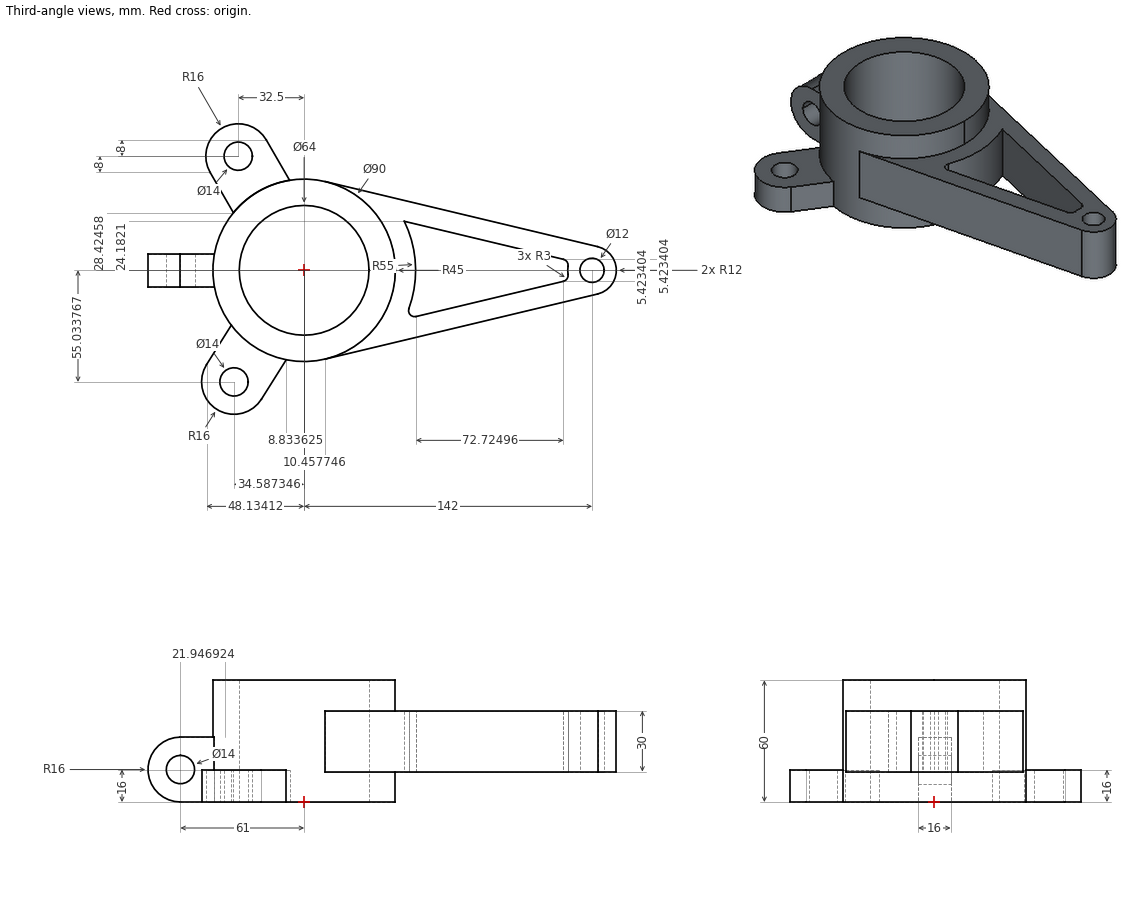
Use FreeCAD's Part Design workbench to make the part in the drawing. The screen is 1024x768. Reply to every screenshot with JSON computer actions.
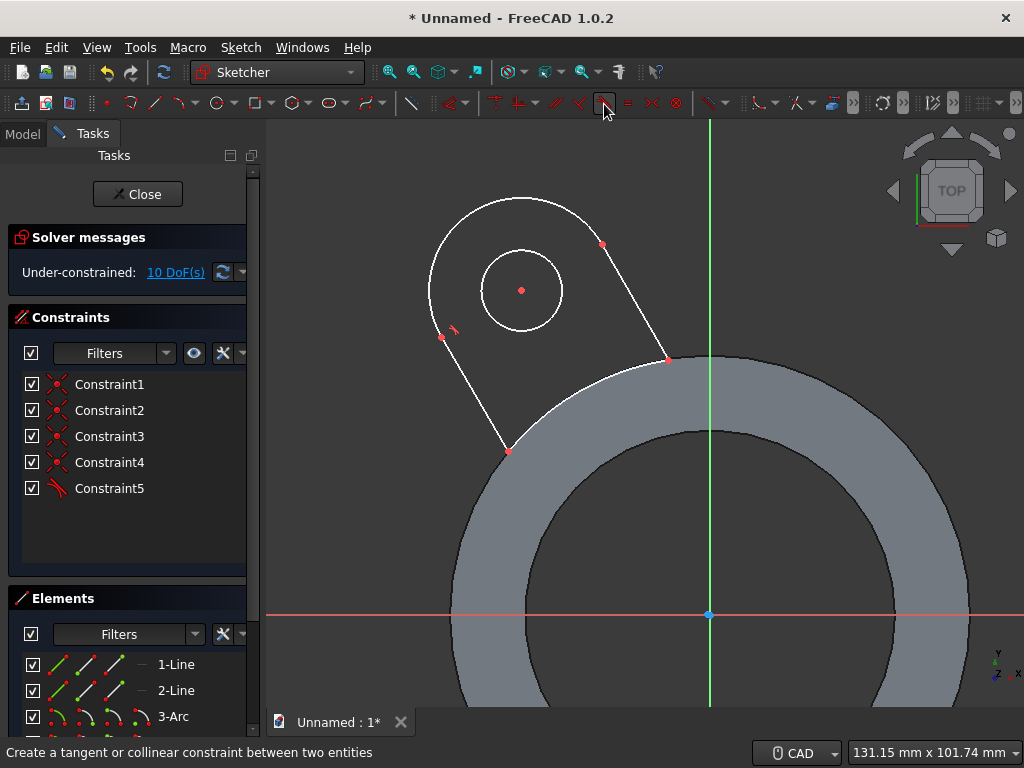
{"action": "left_click", "coordinate": [649, 325]}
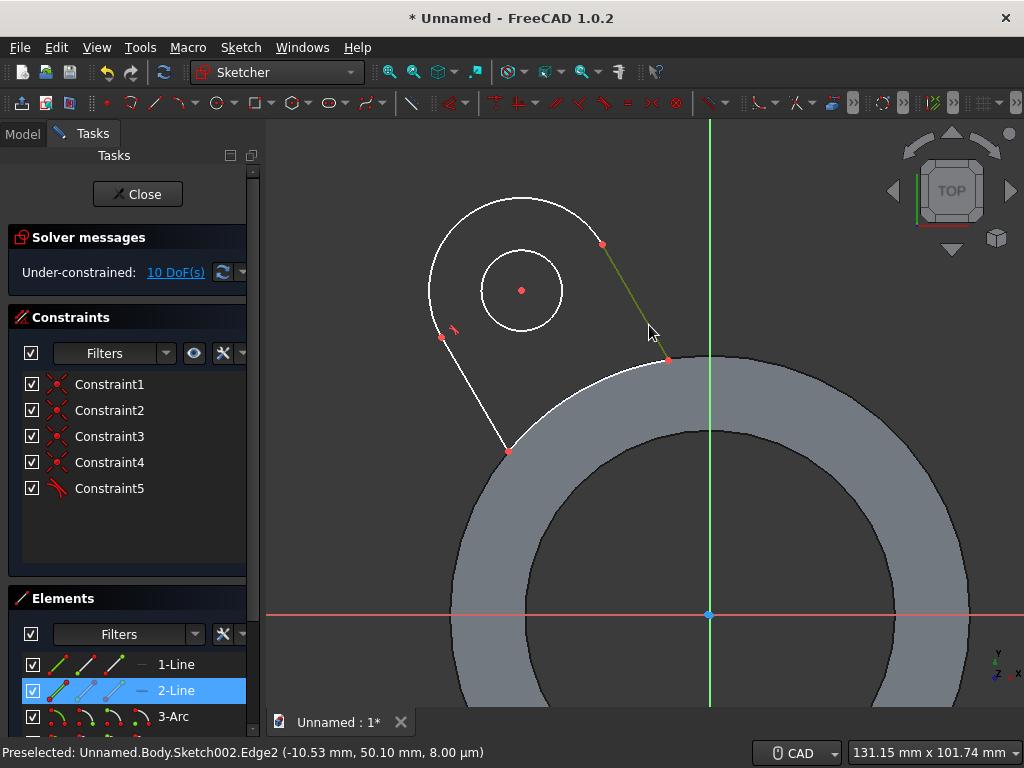
{"action": "left_click", "coordinate": [532, 198]}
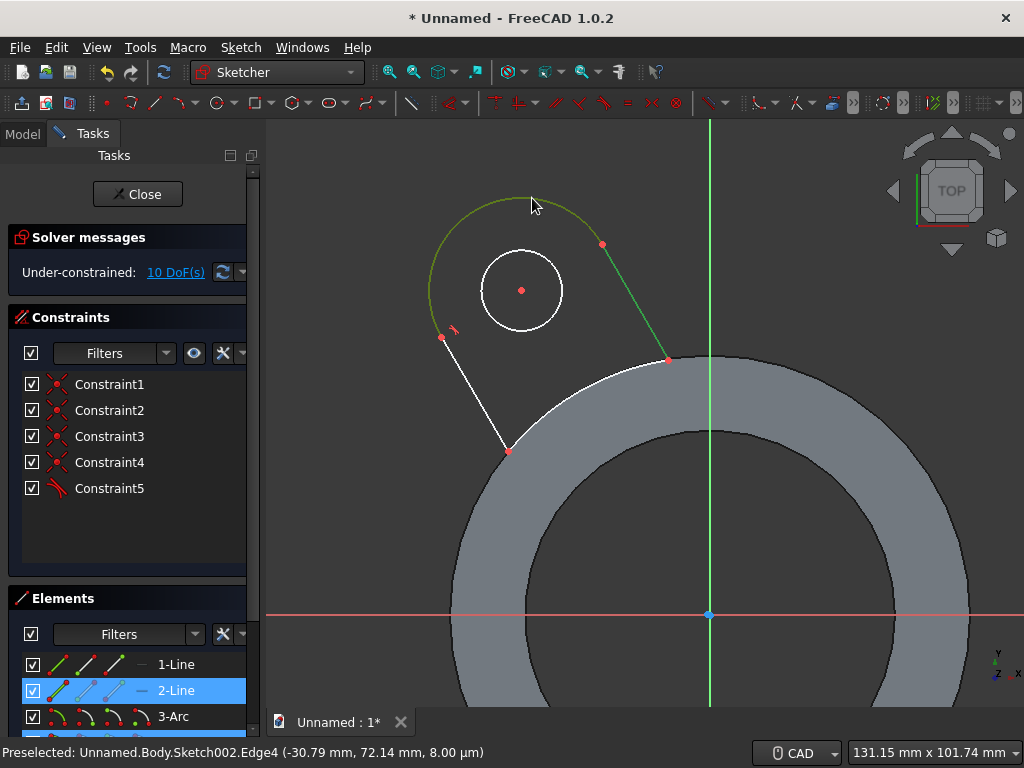
{"action": "key", "text": "t"}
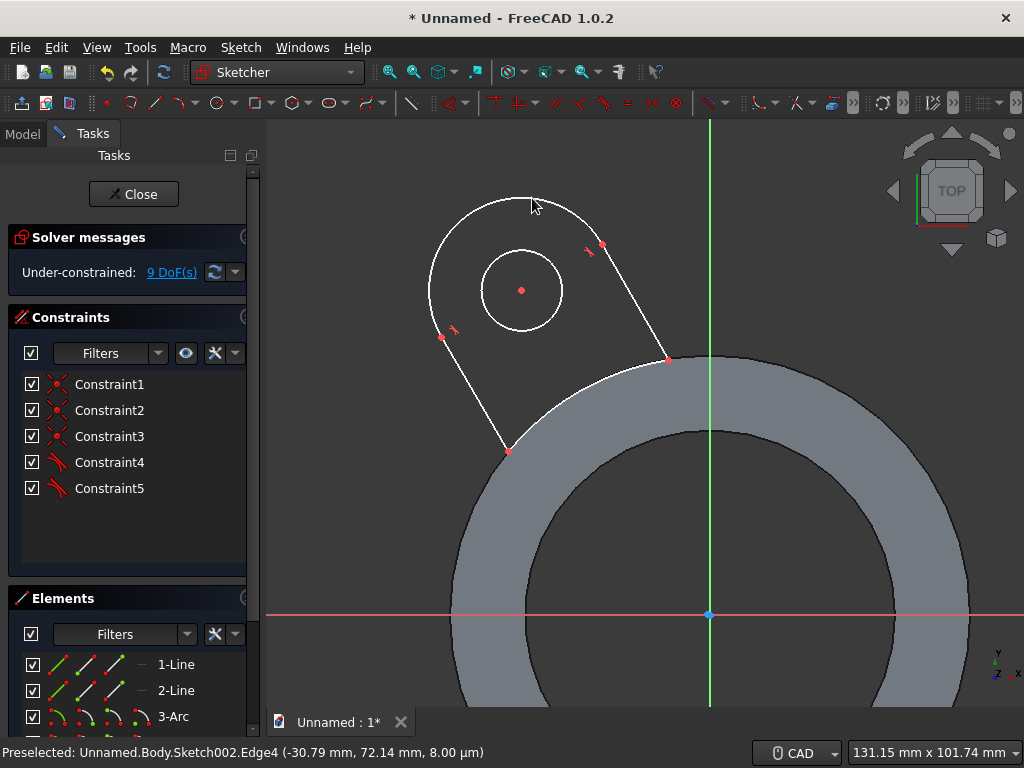
{"action": "left_click_drag", "start_coordinate": [698, 604], "coordinate": [720, 625]}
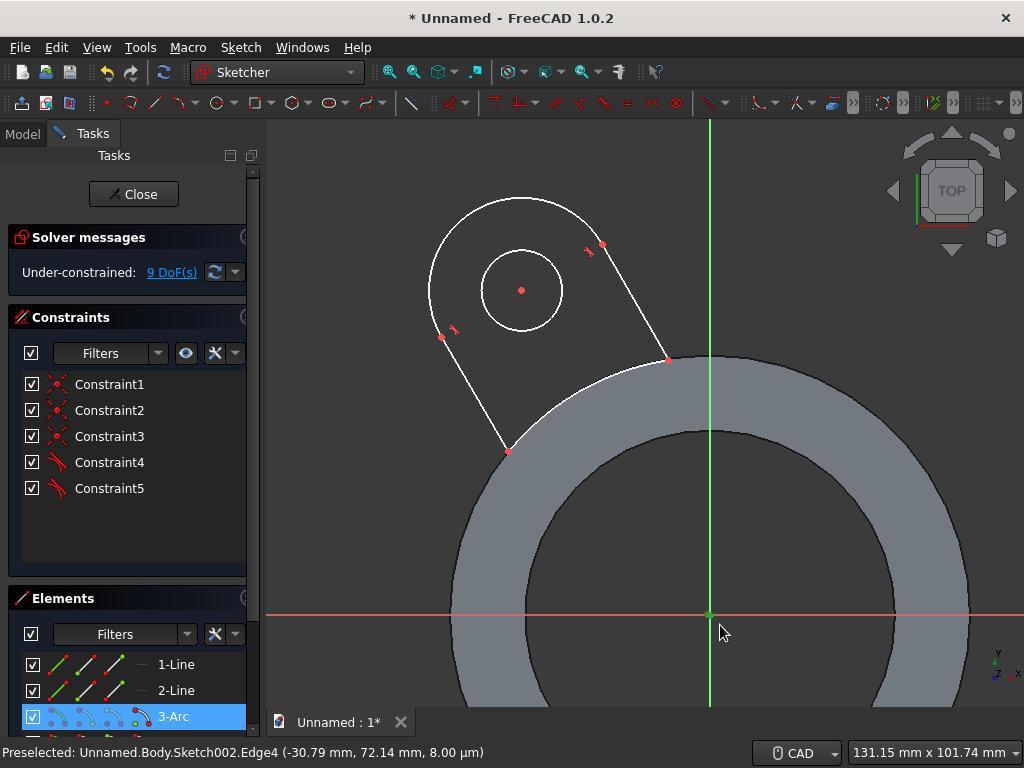
{"action": "left_click", "coordinate": [496, 104]}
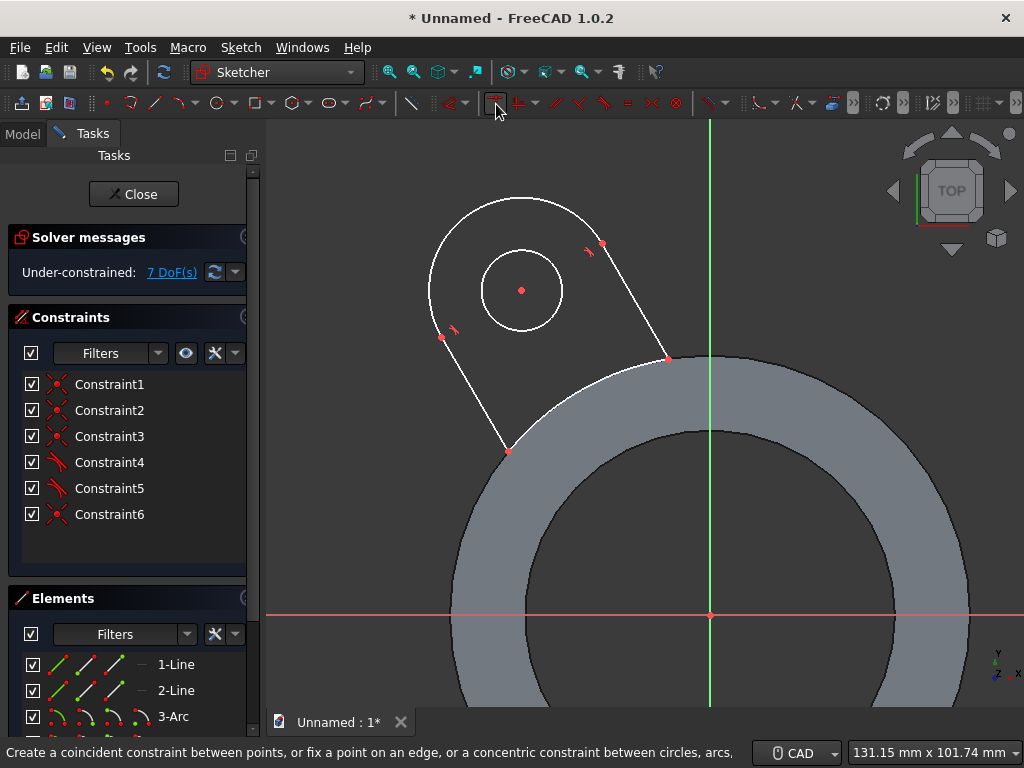
{"action": "left_click", "coordinate": [450, 104]}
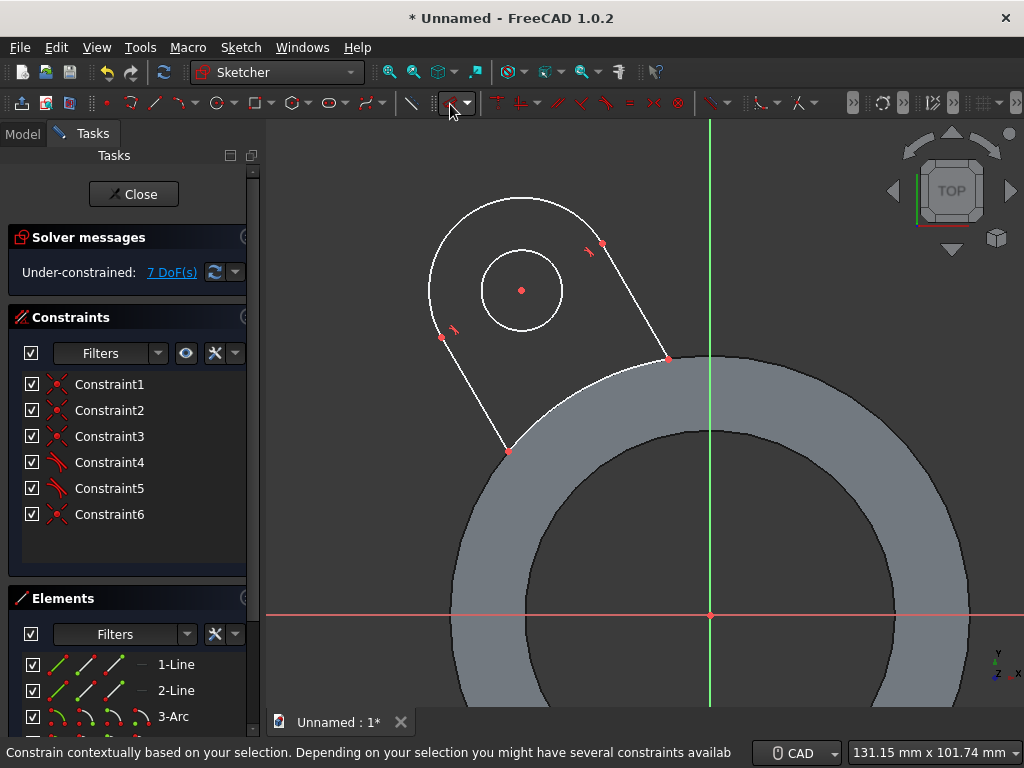
{"action": "left_click", "coordinate": [614, 374]}
{"action": "left_click", "coordinate": [602, 344]}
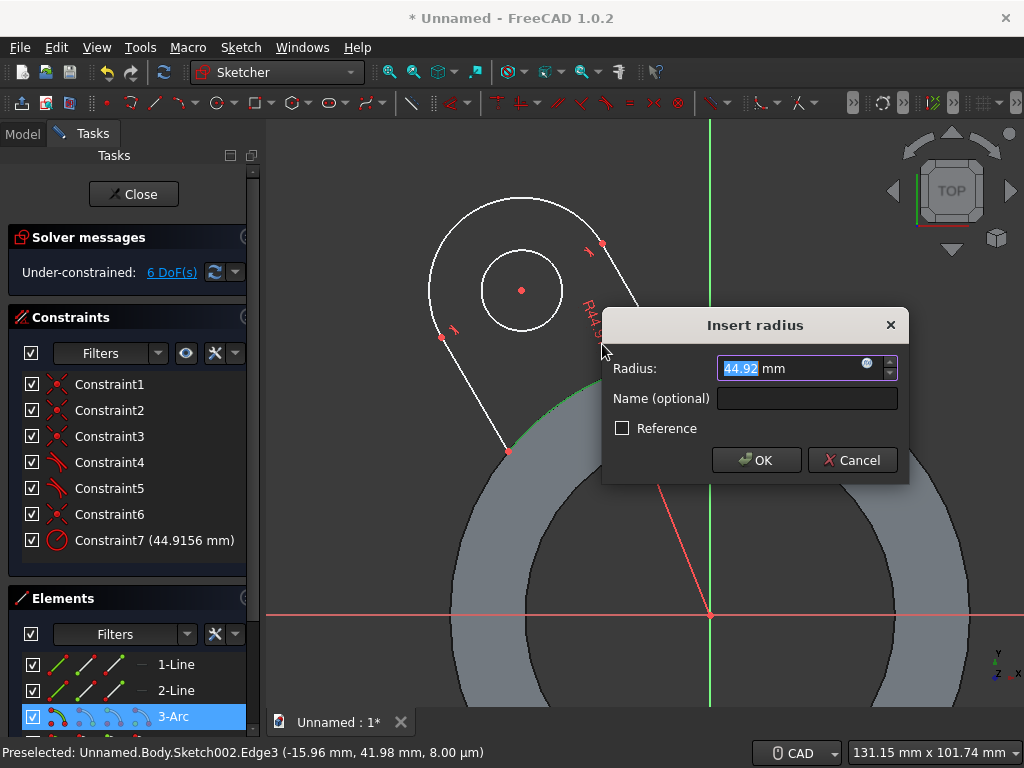
{"action": "type", "text": "45"}
{"action": "key", "text": "Return"}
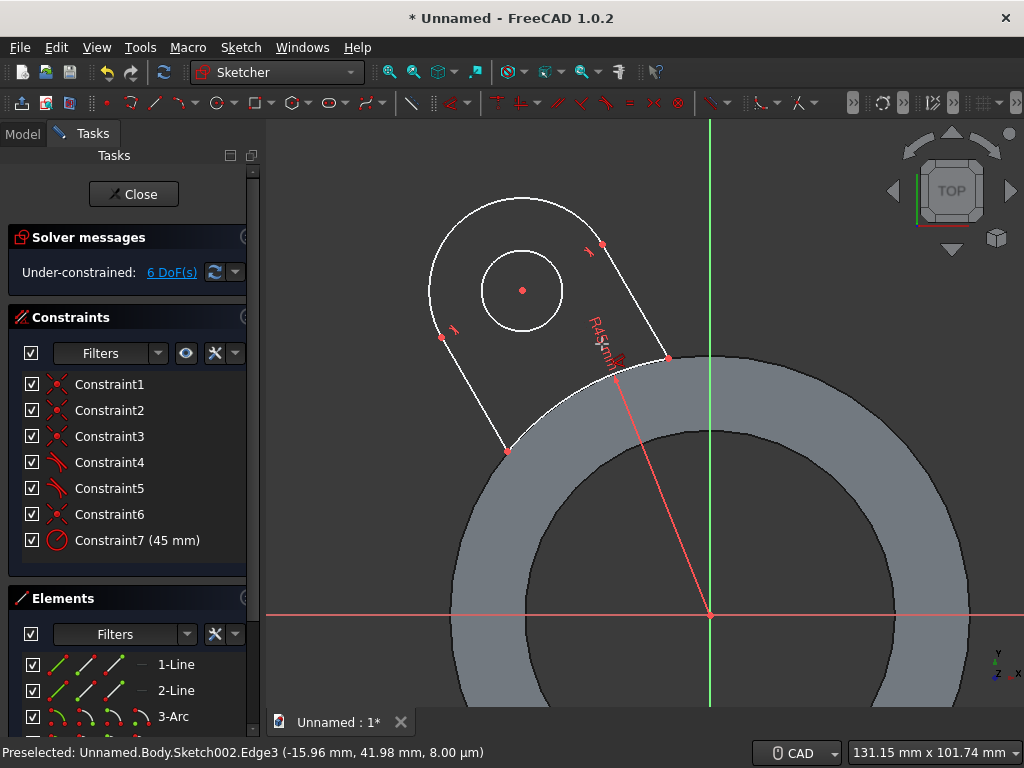
{"action": "left_click", "coordinate": [531, 199]}
{"action": "left_click", "coordinate": [534, 167]}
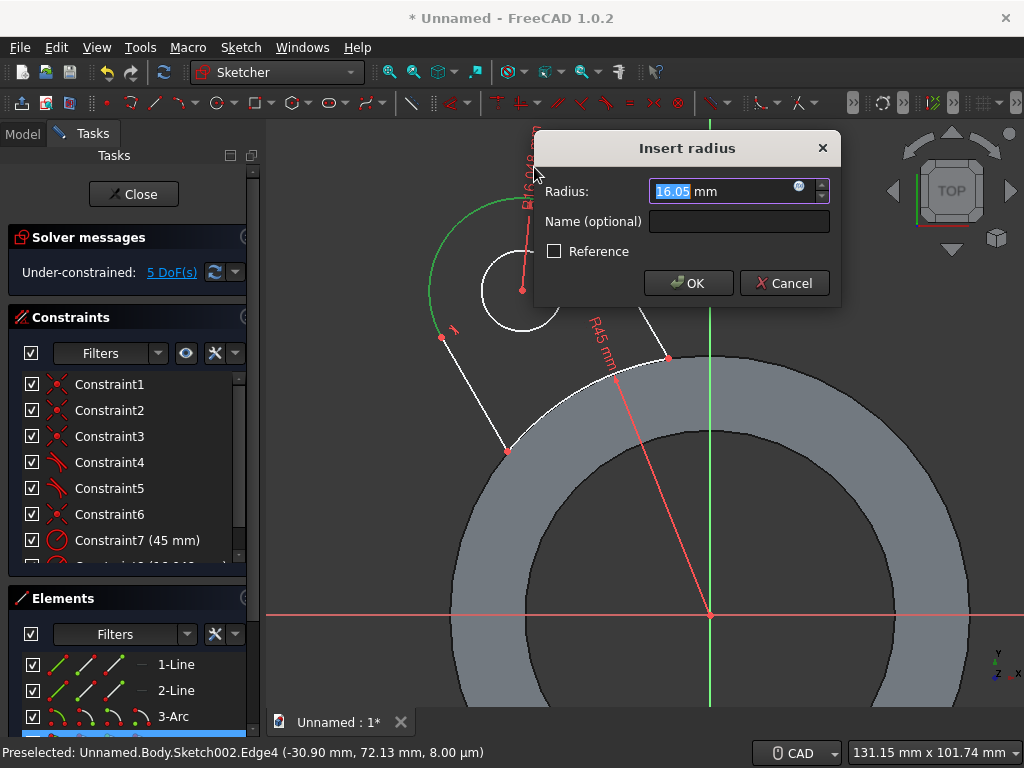
{"action": "type", "text": "16"}
{"action": "key", "text": "Return"}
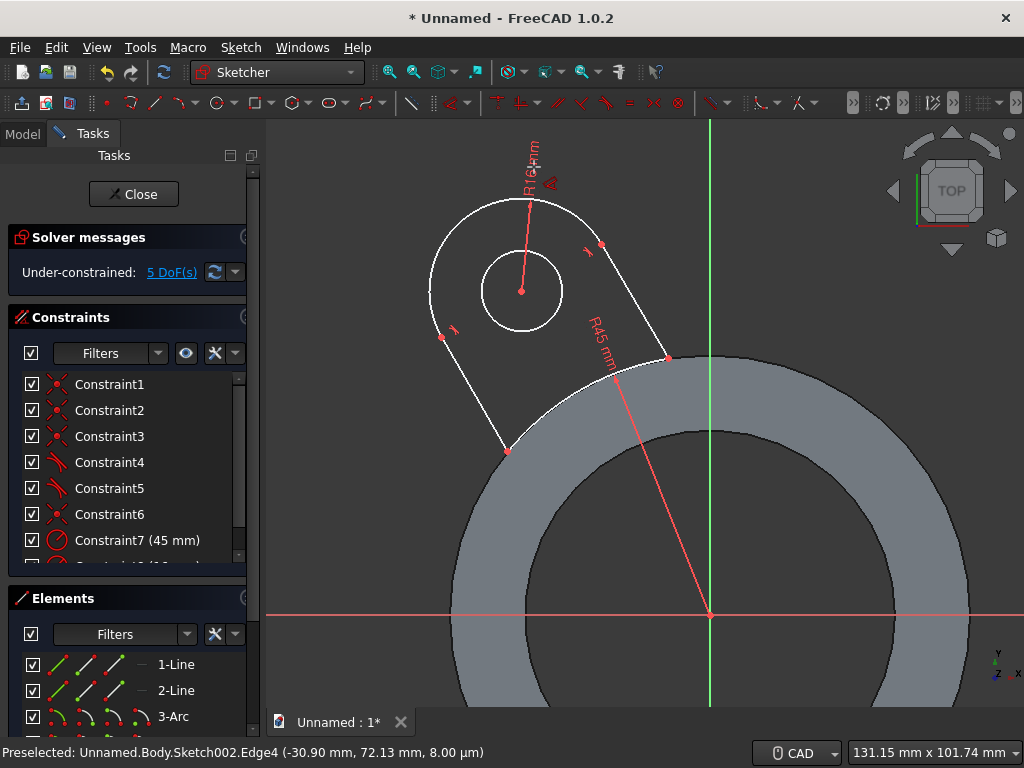
{"action": "left_click", "coordinate": [550, 263]}
{"action": "left_click", "coordinate": [573, 240]}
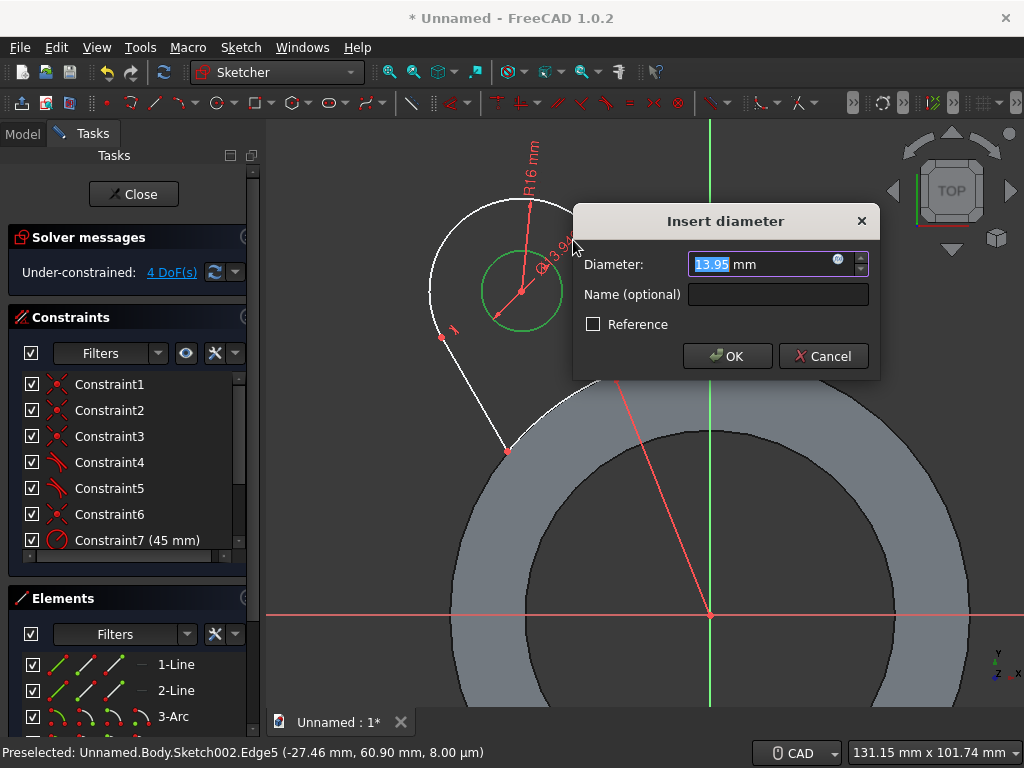
{"action": "type", "text": "14"}
{"action": "key", "text": "Return"}